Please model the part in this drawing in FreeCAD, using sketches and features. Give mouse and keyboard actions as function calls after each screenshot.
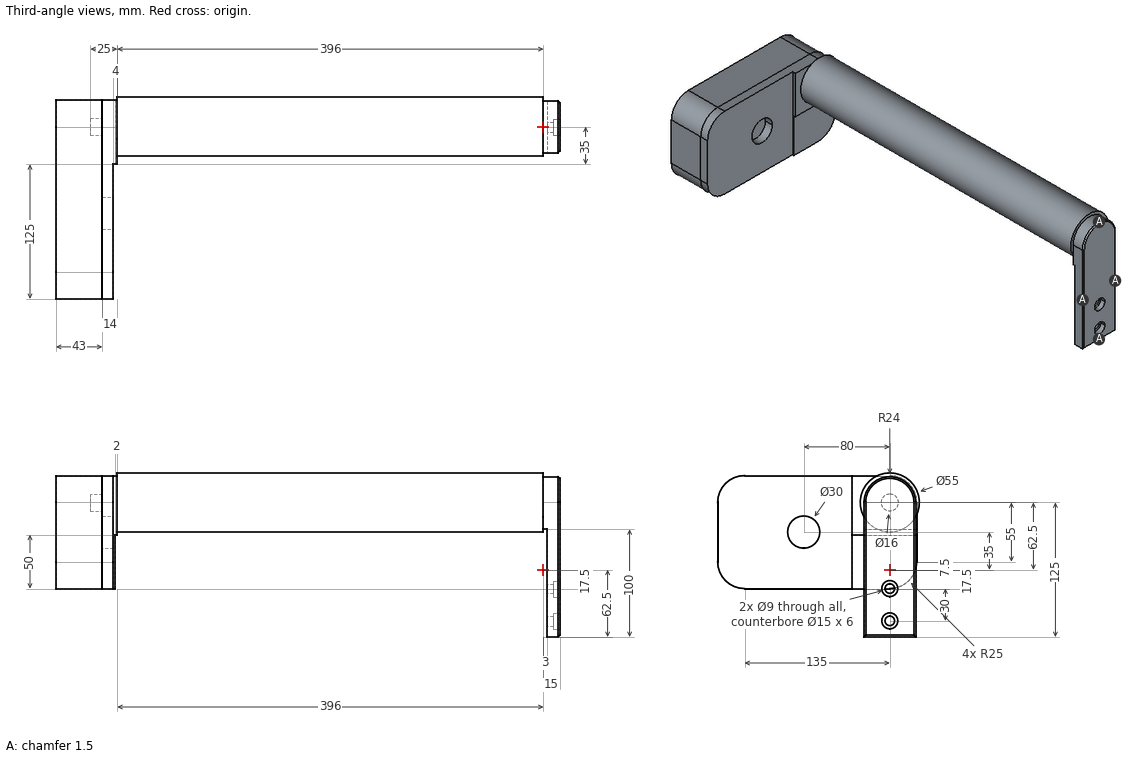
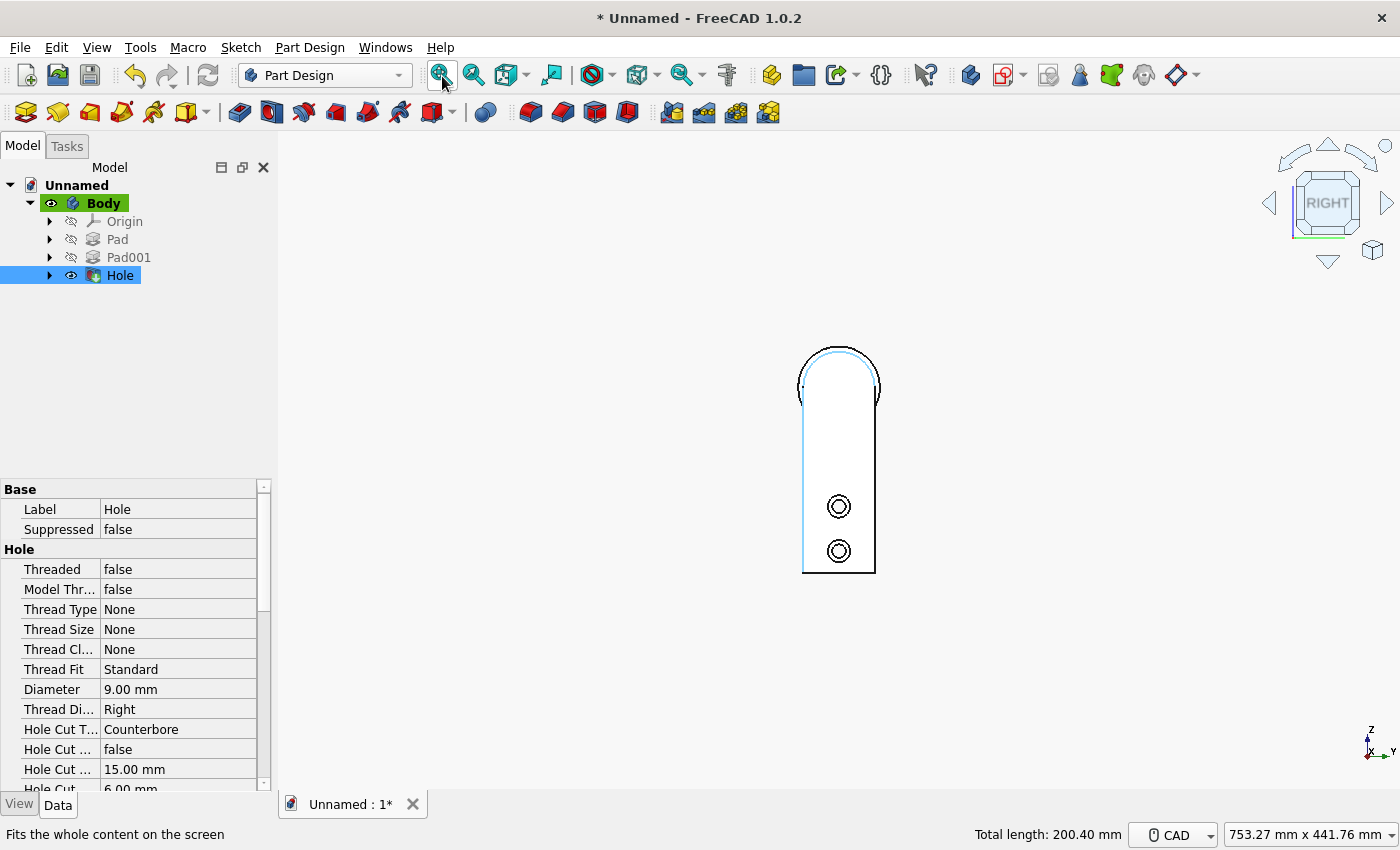
click(839, 572, ctrl)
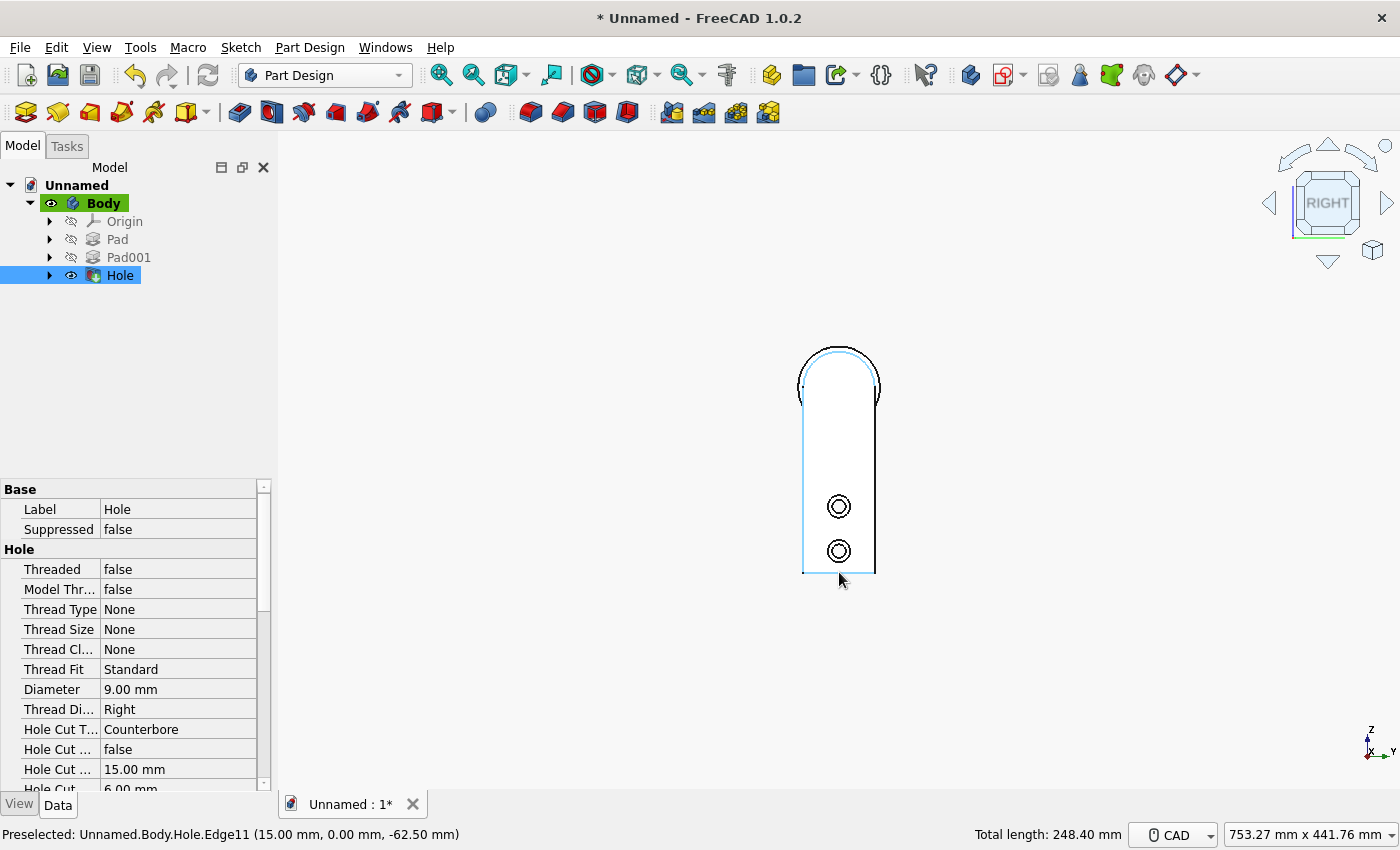
click(875, 479, ctrl)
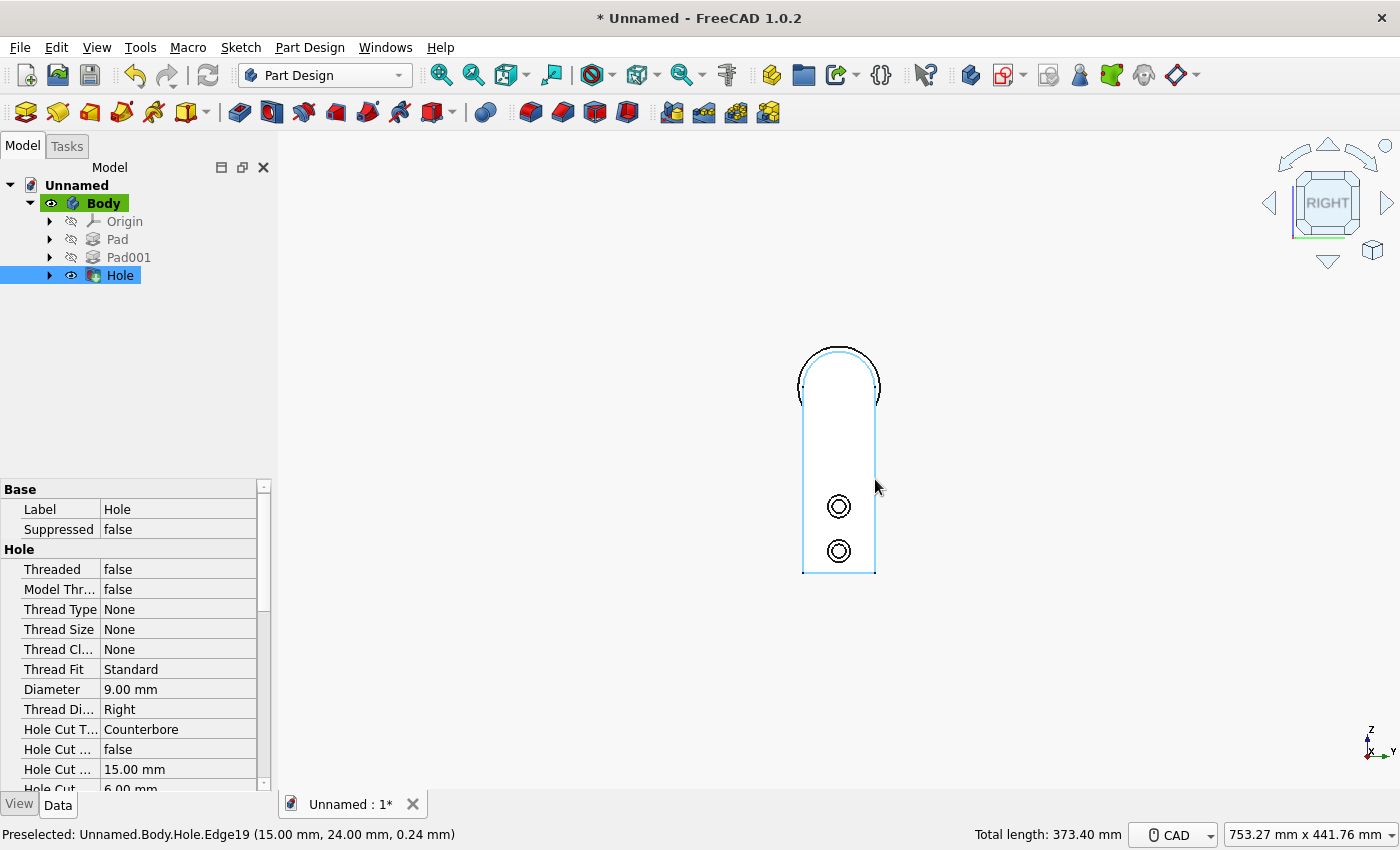
click(564, 112)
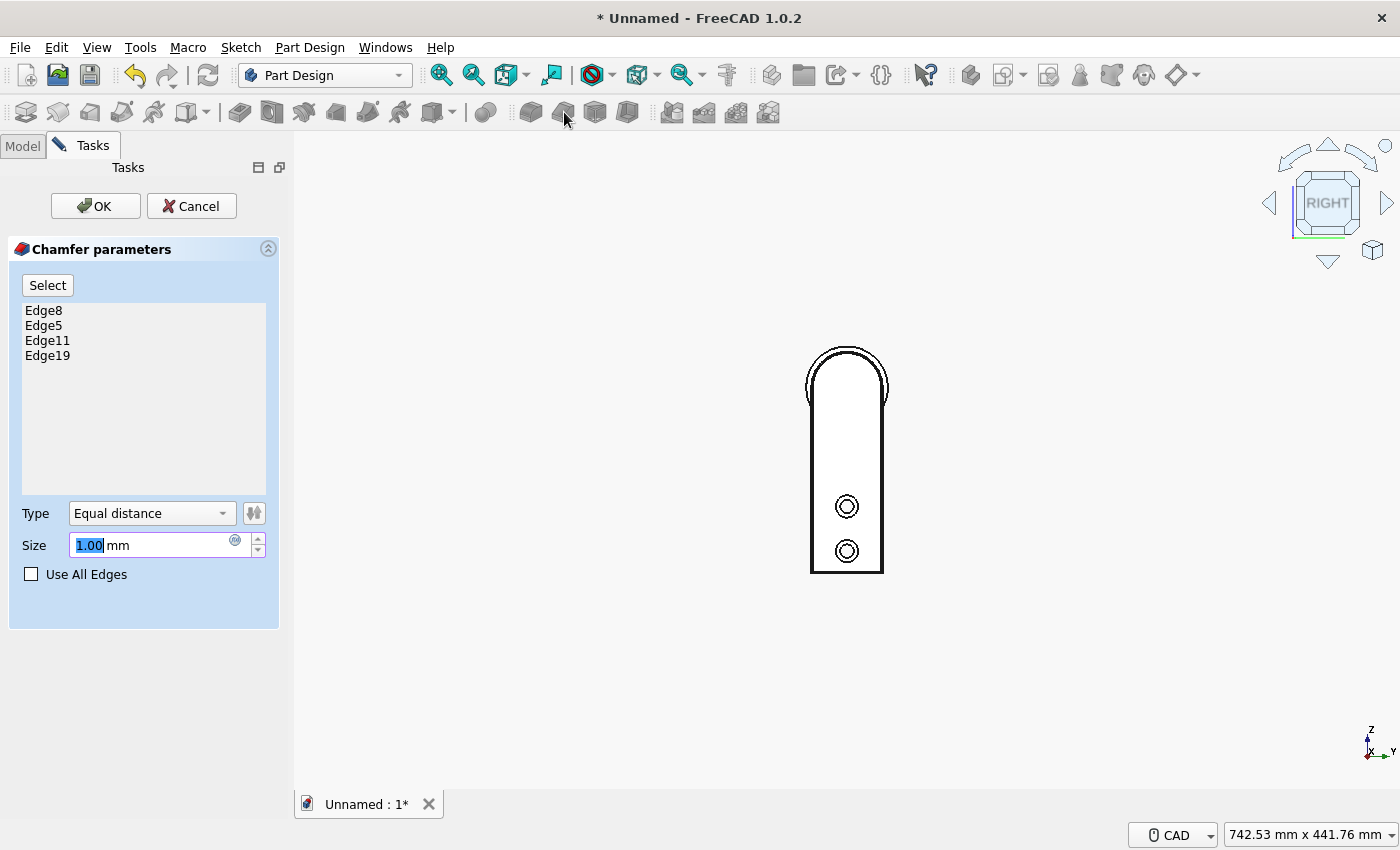
text(1.5)
key(Tab)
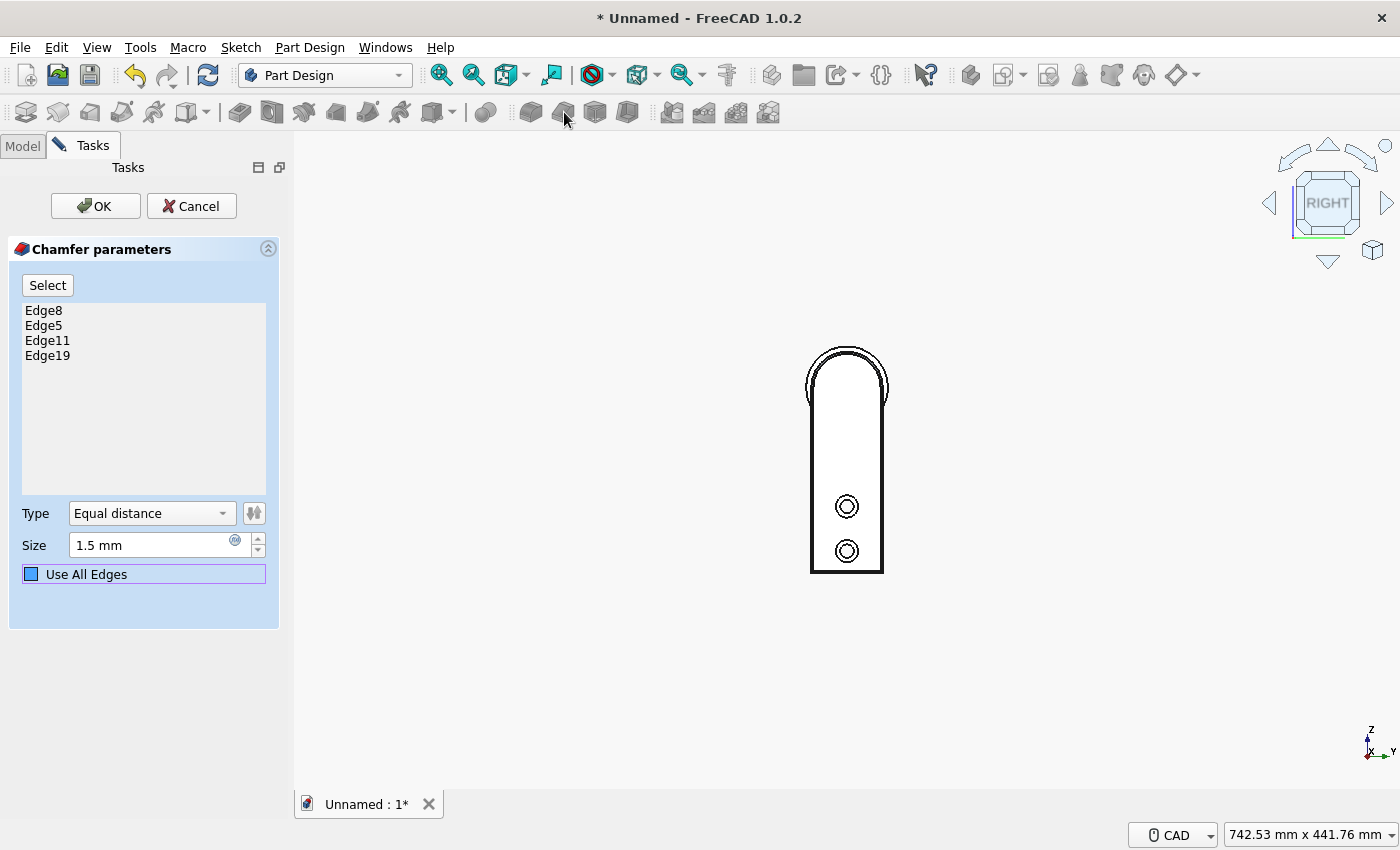
click(96, 206)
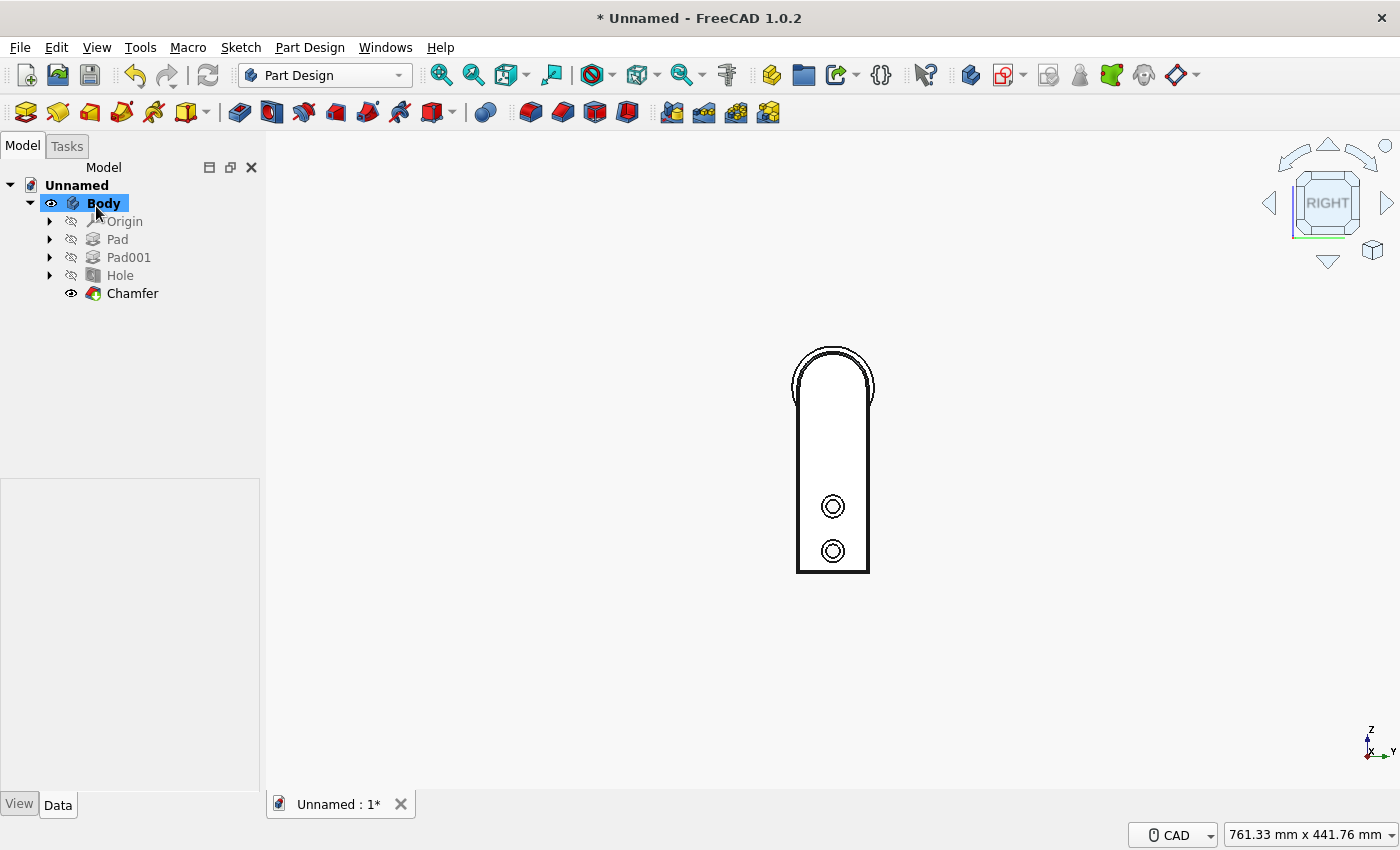
key(v)
key(f)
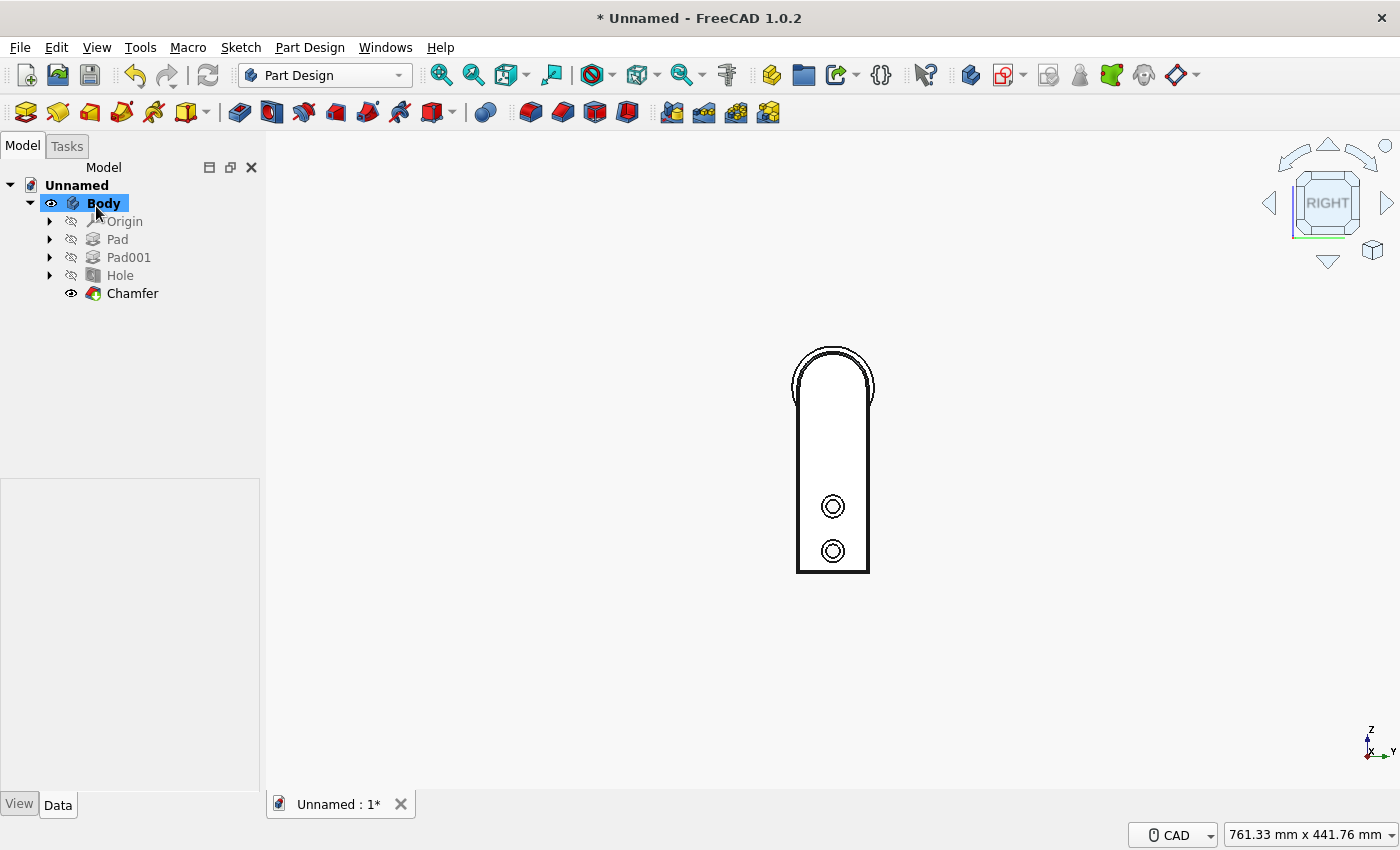
key(4)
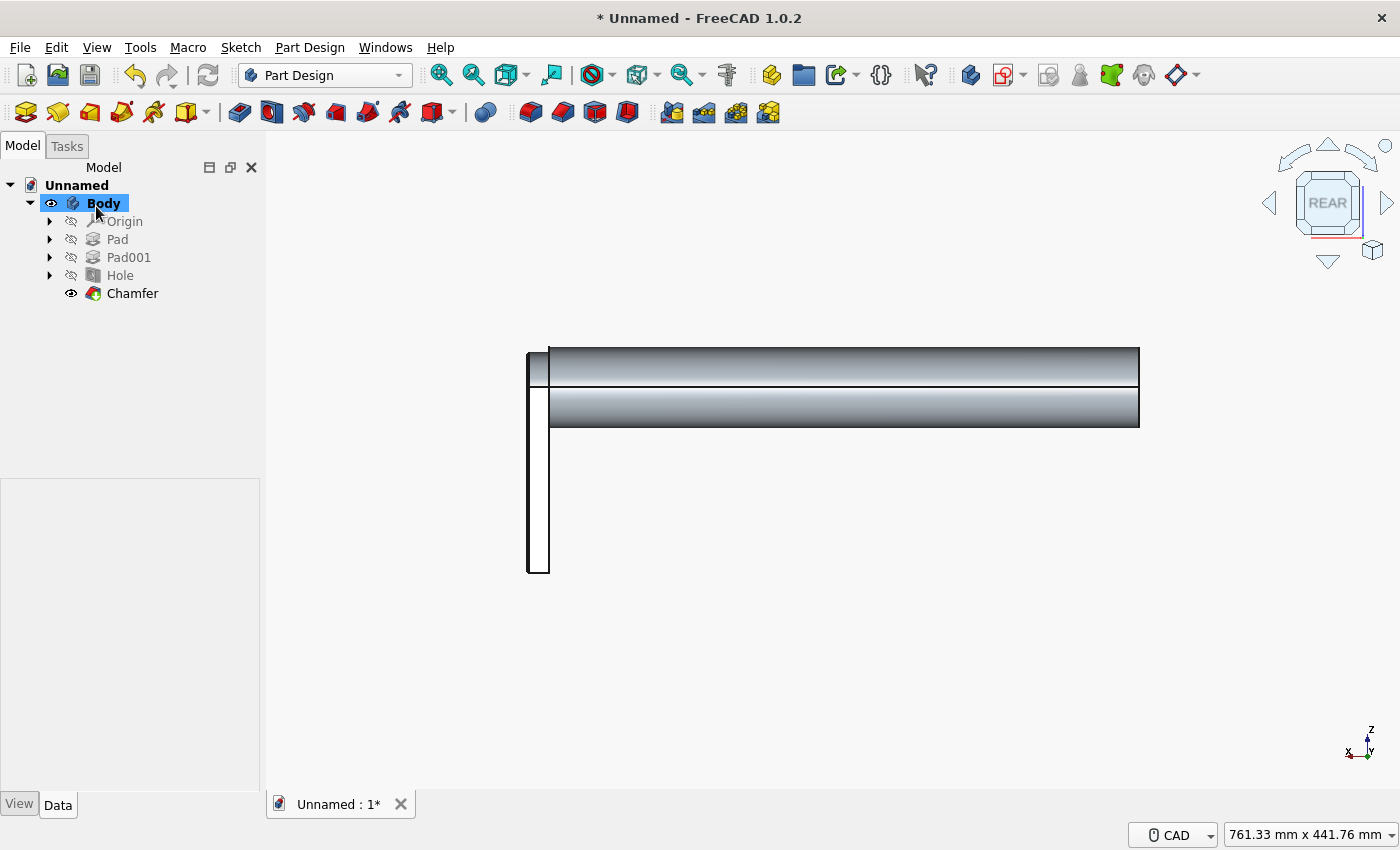
click(539, 533)